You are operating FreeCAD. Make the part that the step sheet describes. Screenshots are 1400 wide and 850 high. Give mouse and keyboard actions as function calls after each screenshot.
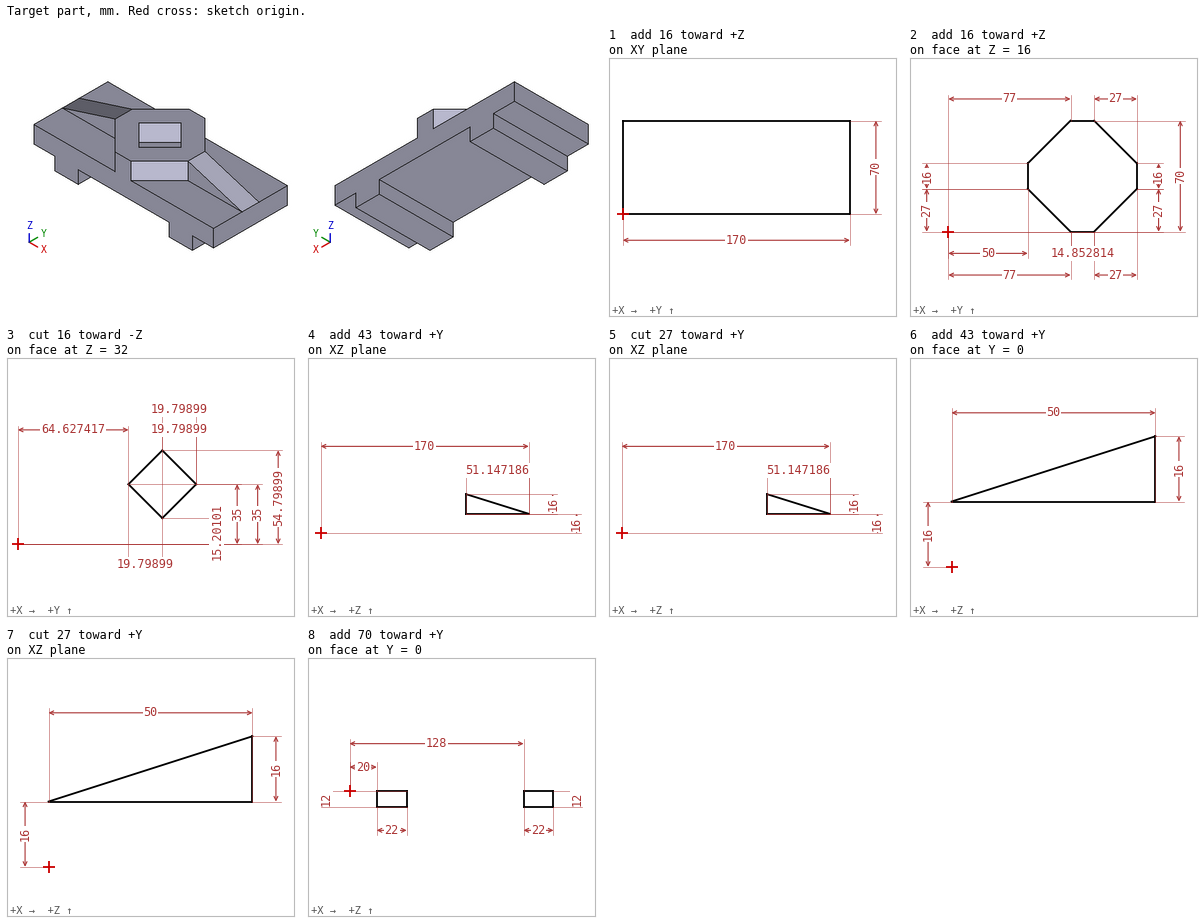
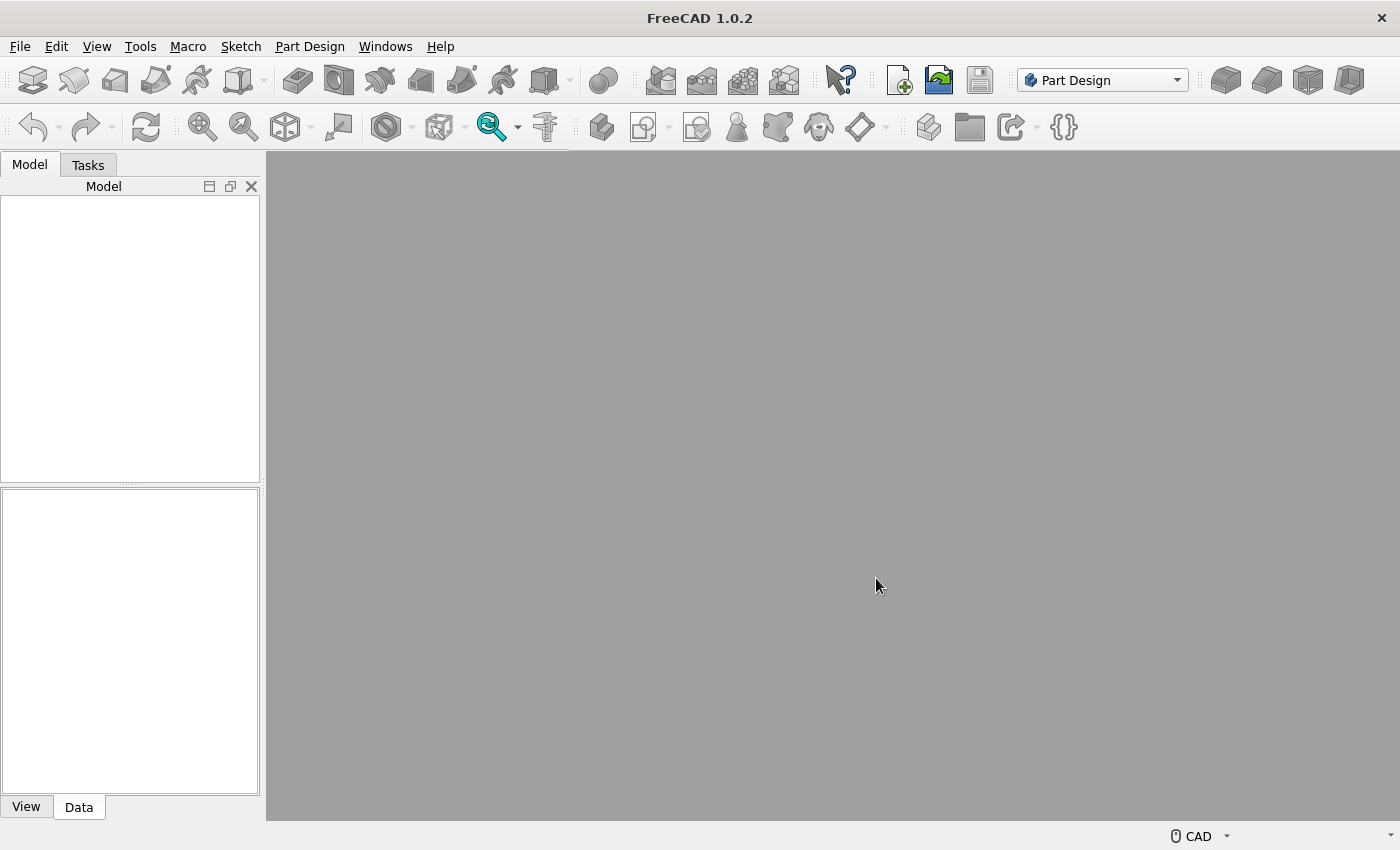
key(ctrl+n)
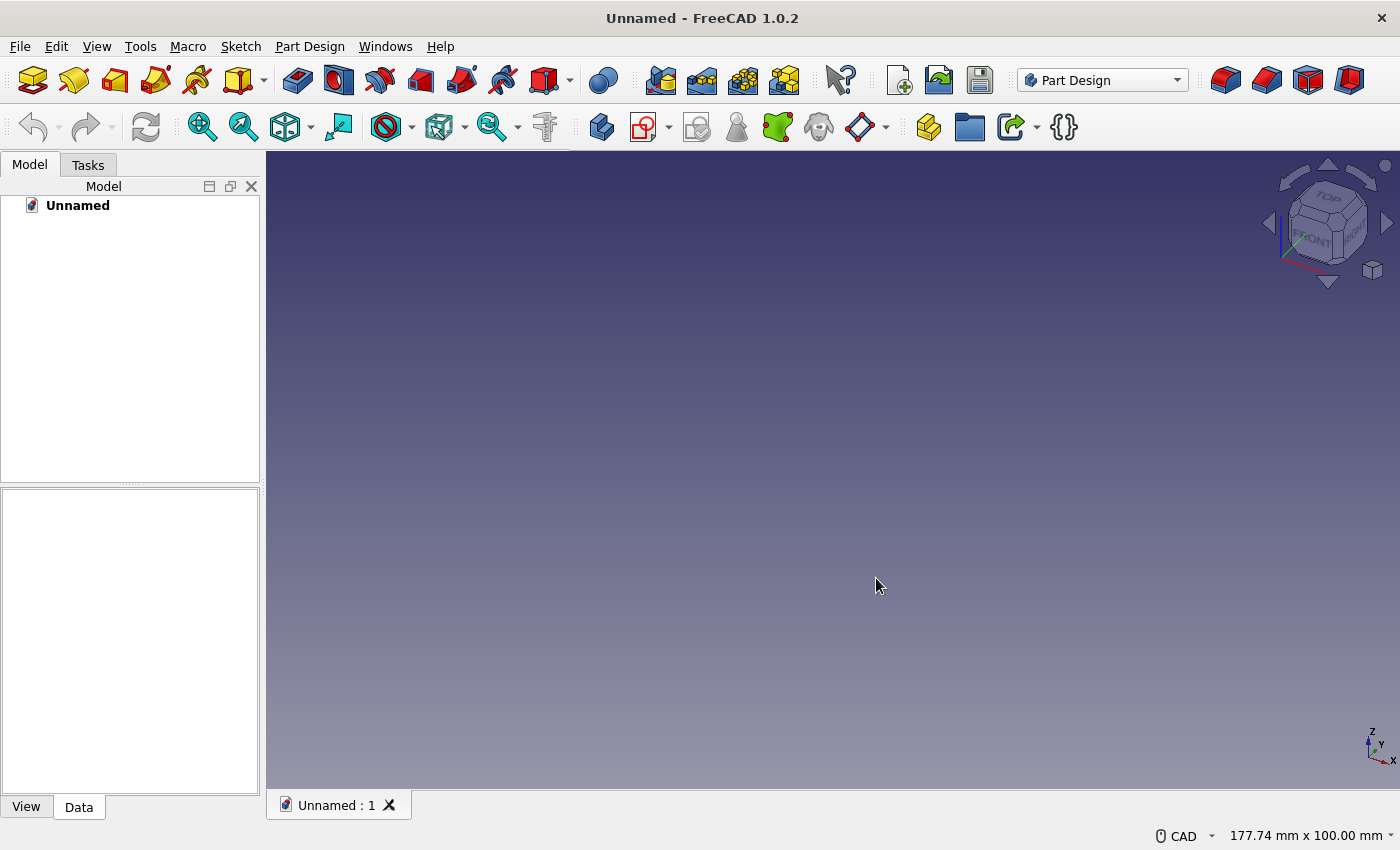
click(642, 128)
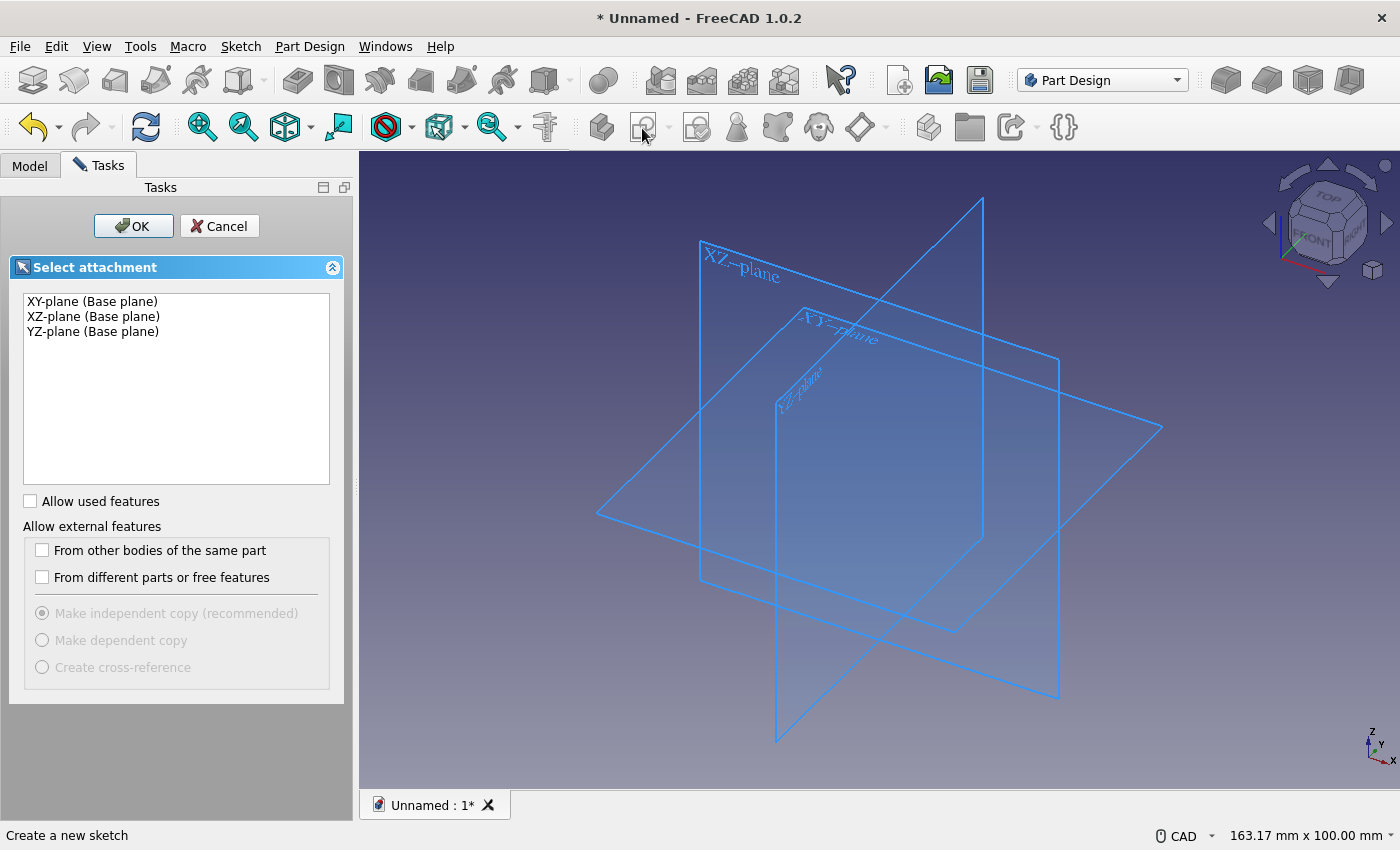
click(84, 302)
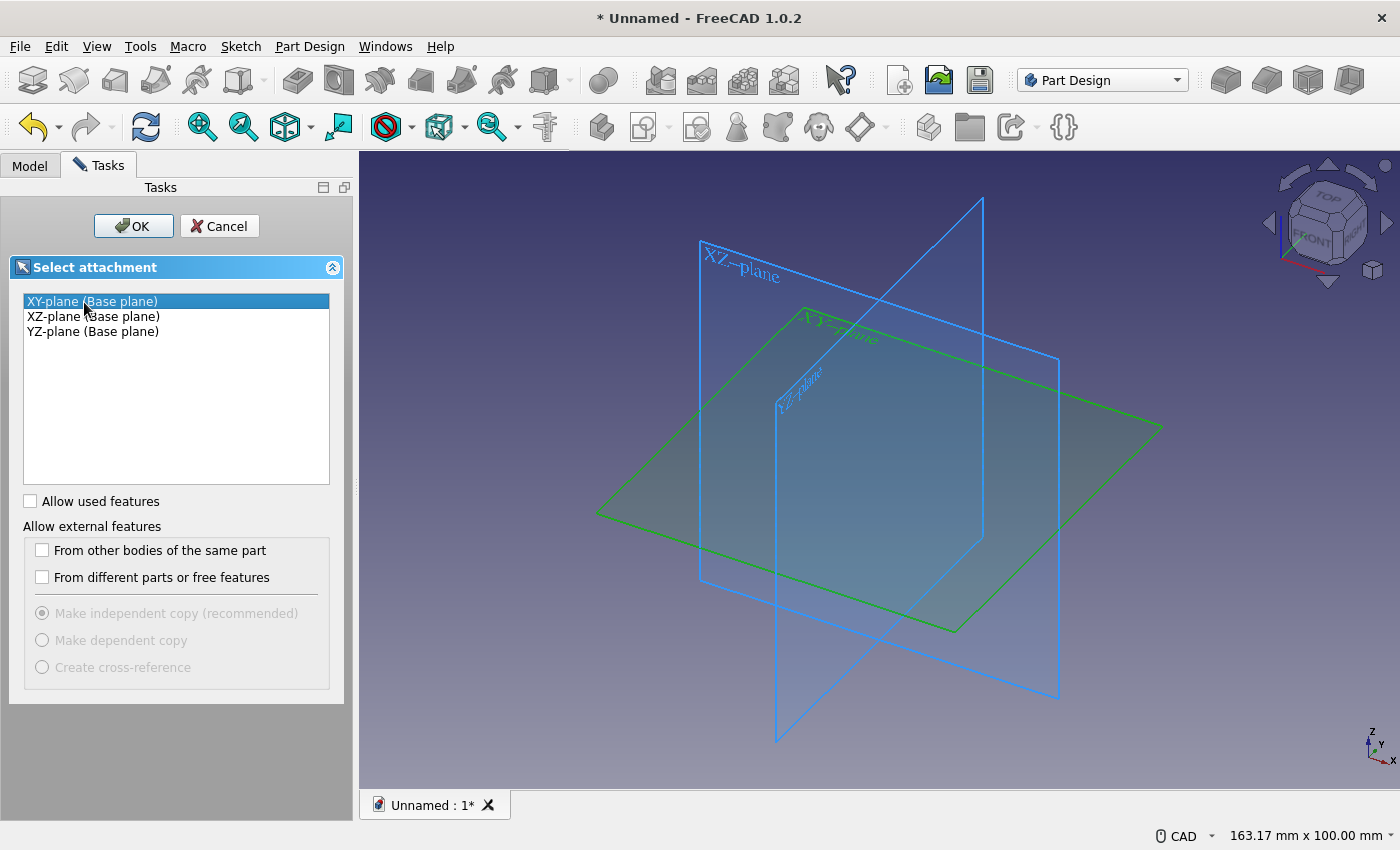
click(134, 226)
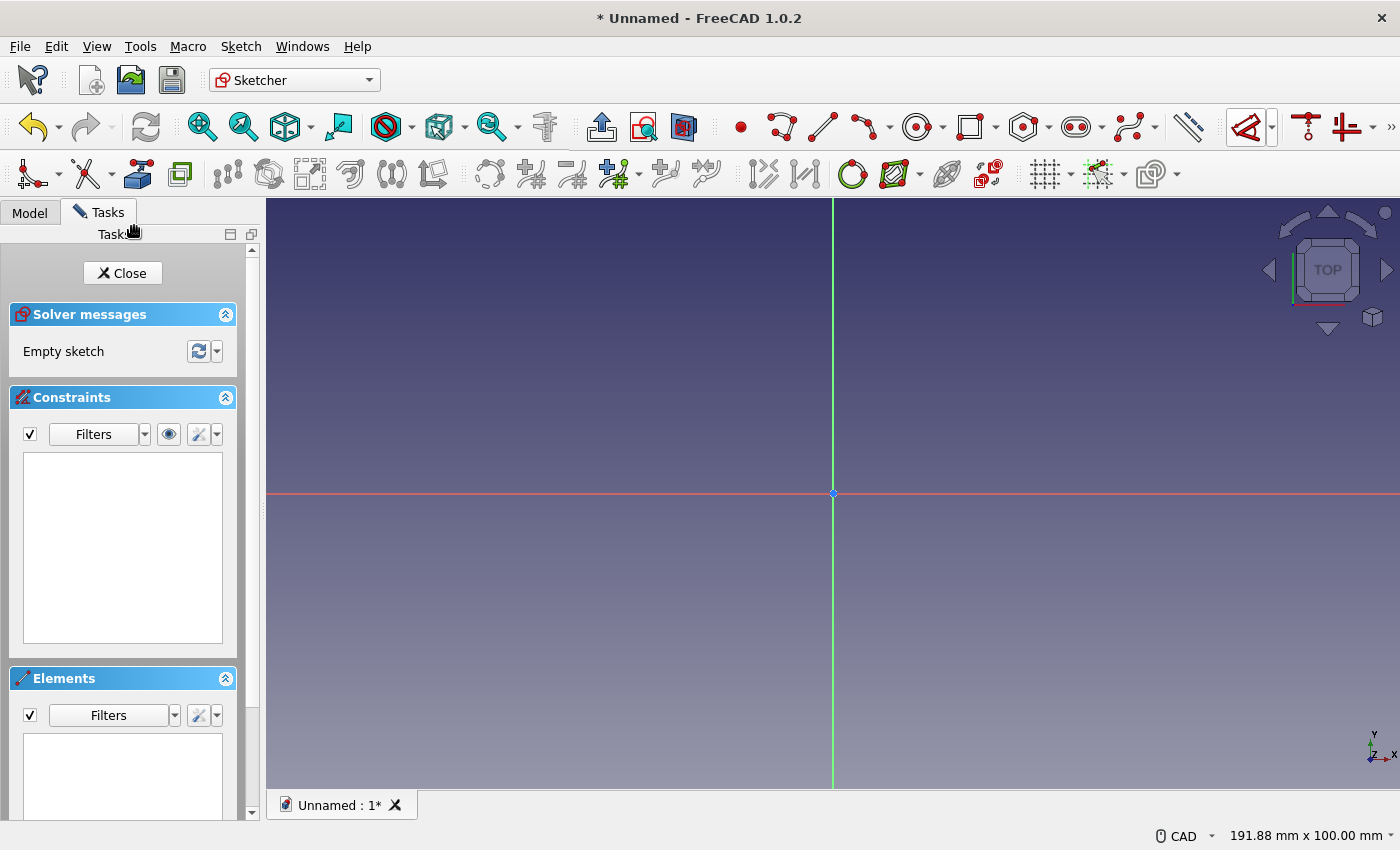
scroll(294, 745, down, 3)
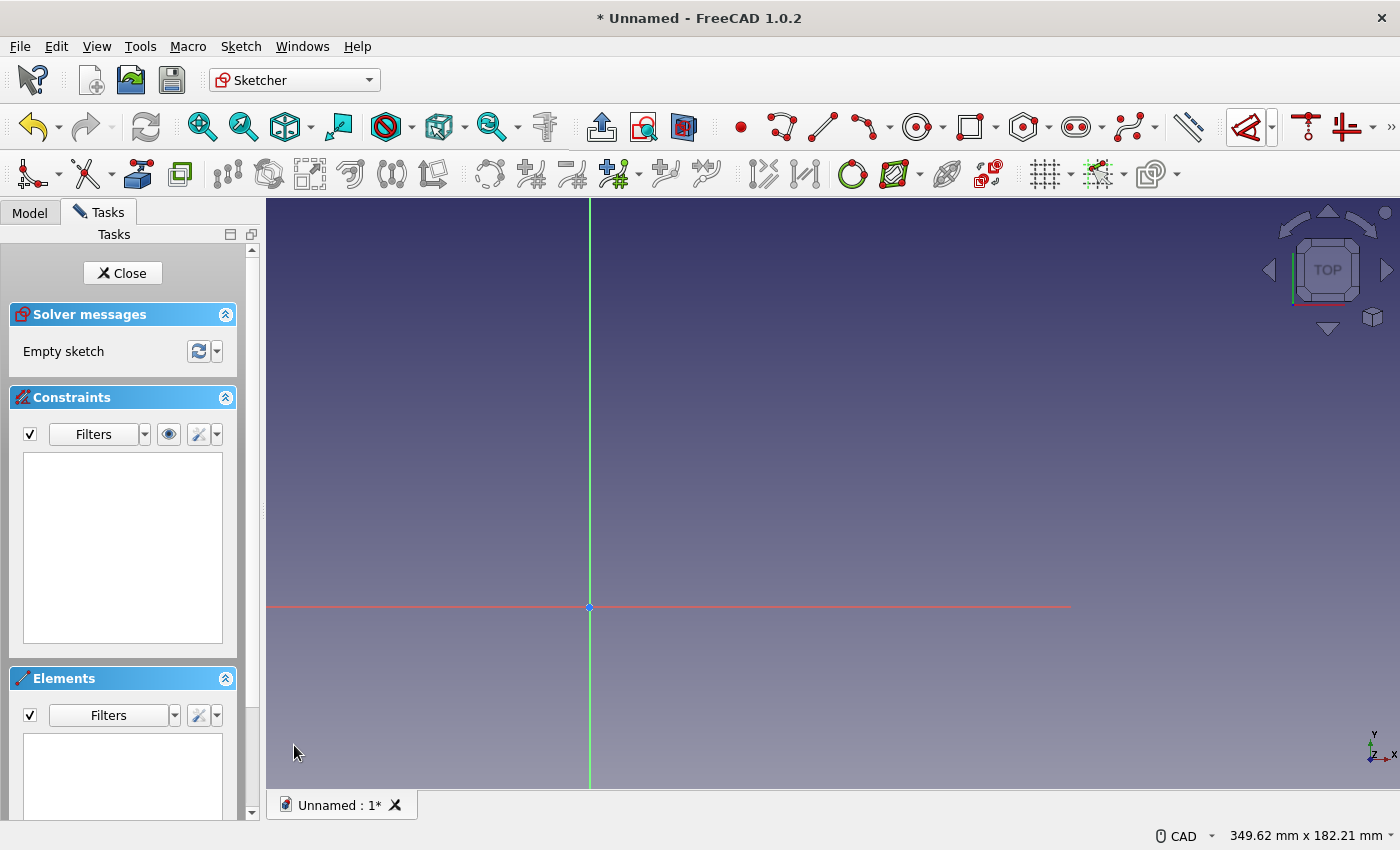
key(g)
key(r)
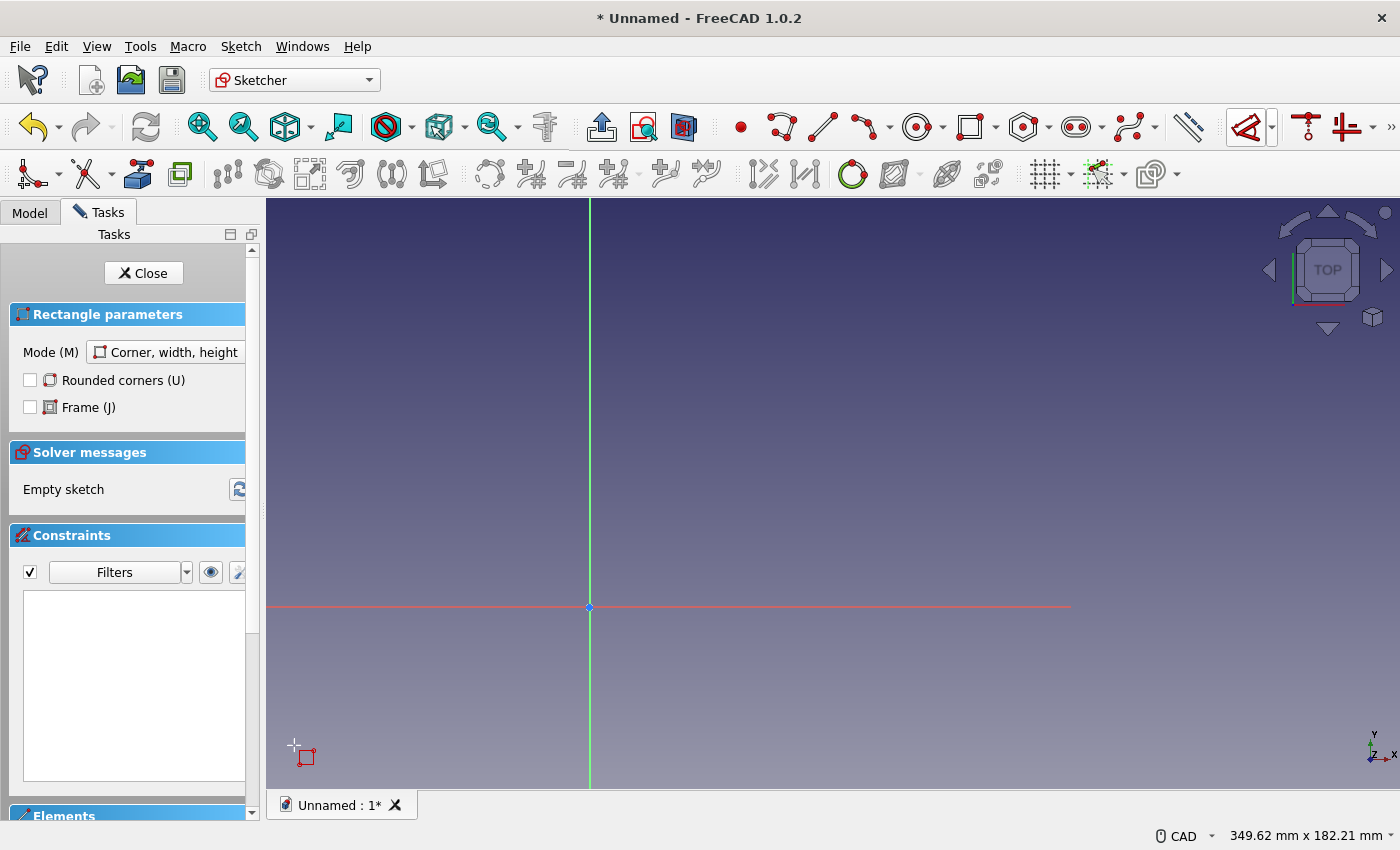
click(590, 607)
move(1141, 380)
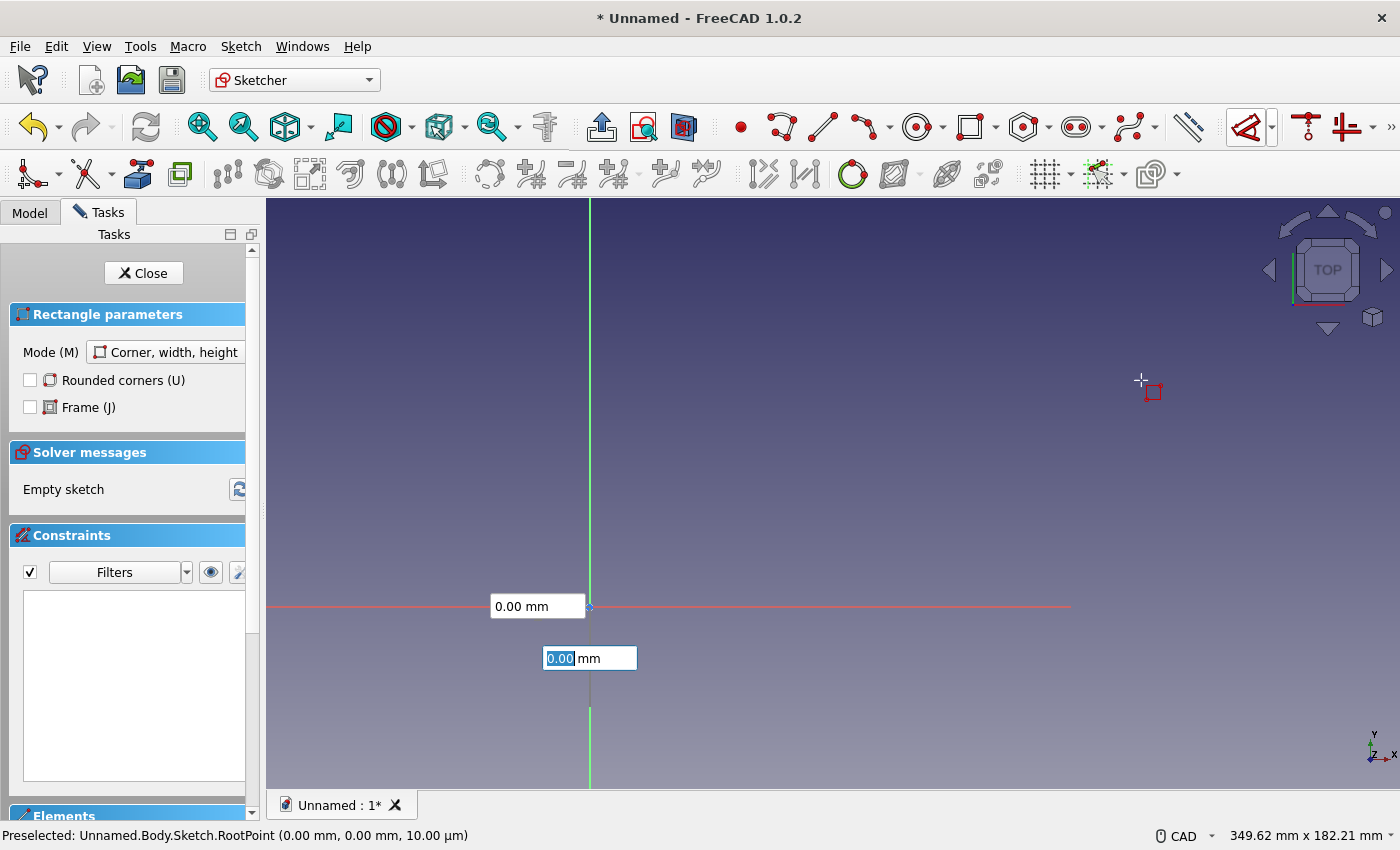
text(170)
key(Tab)
text(70)
key(Return)
key(Escape)